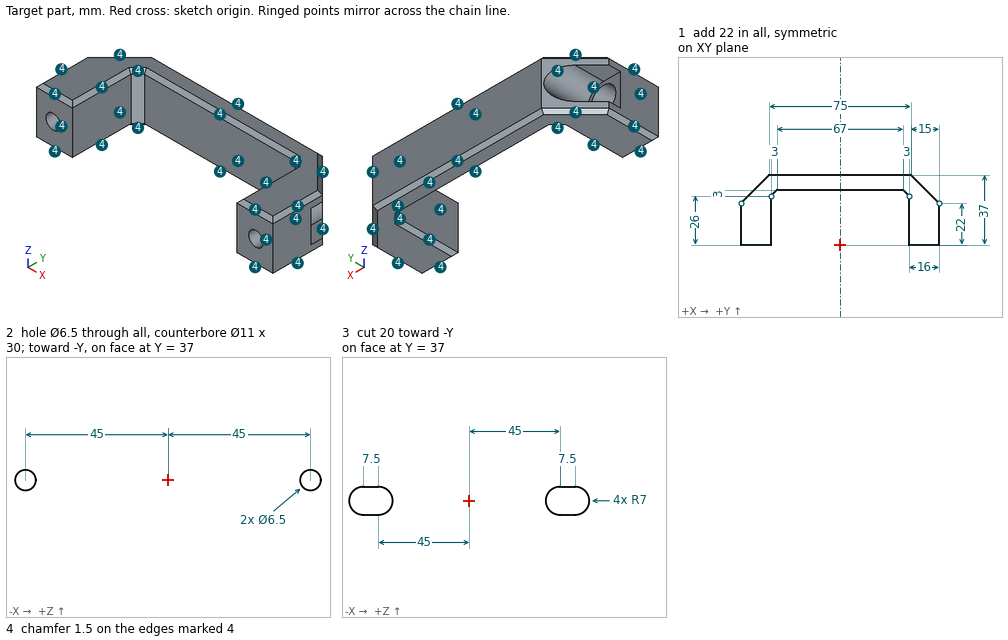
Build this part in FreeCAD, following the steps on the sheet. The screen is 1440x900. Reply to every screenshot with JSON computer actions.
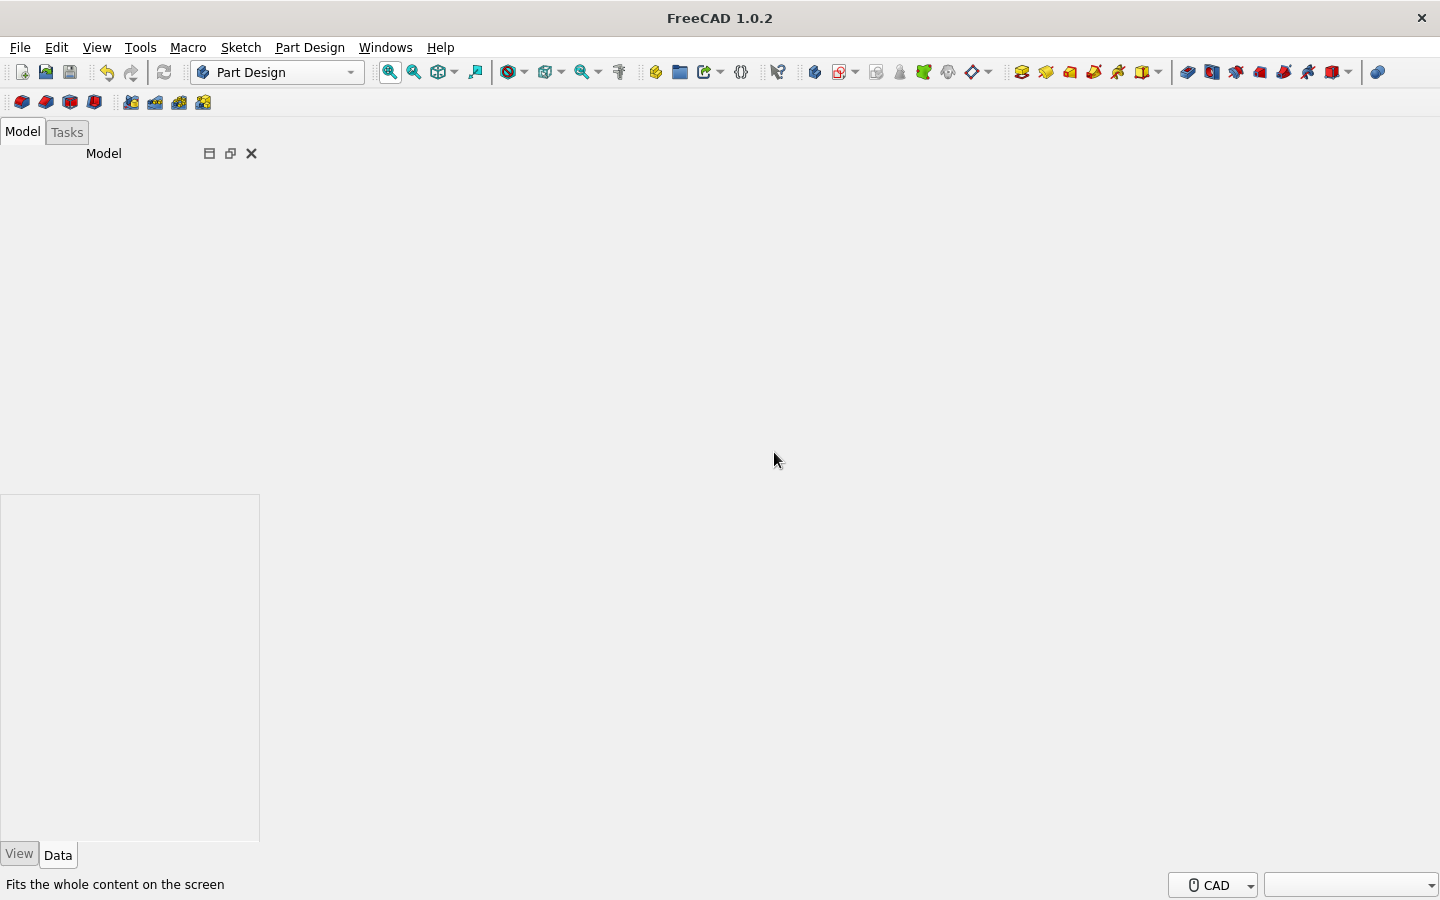
{"action": "left_click", "coordinate": [22, 72]}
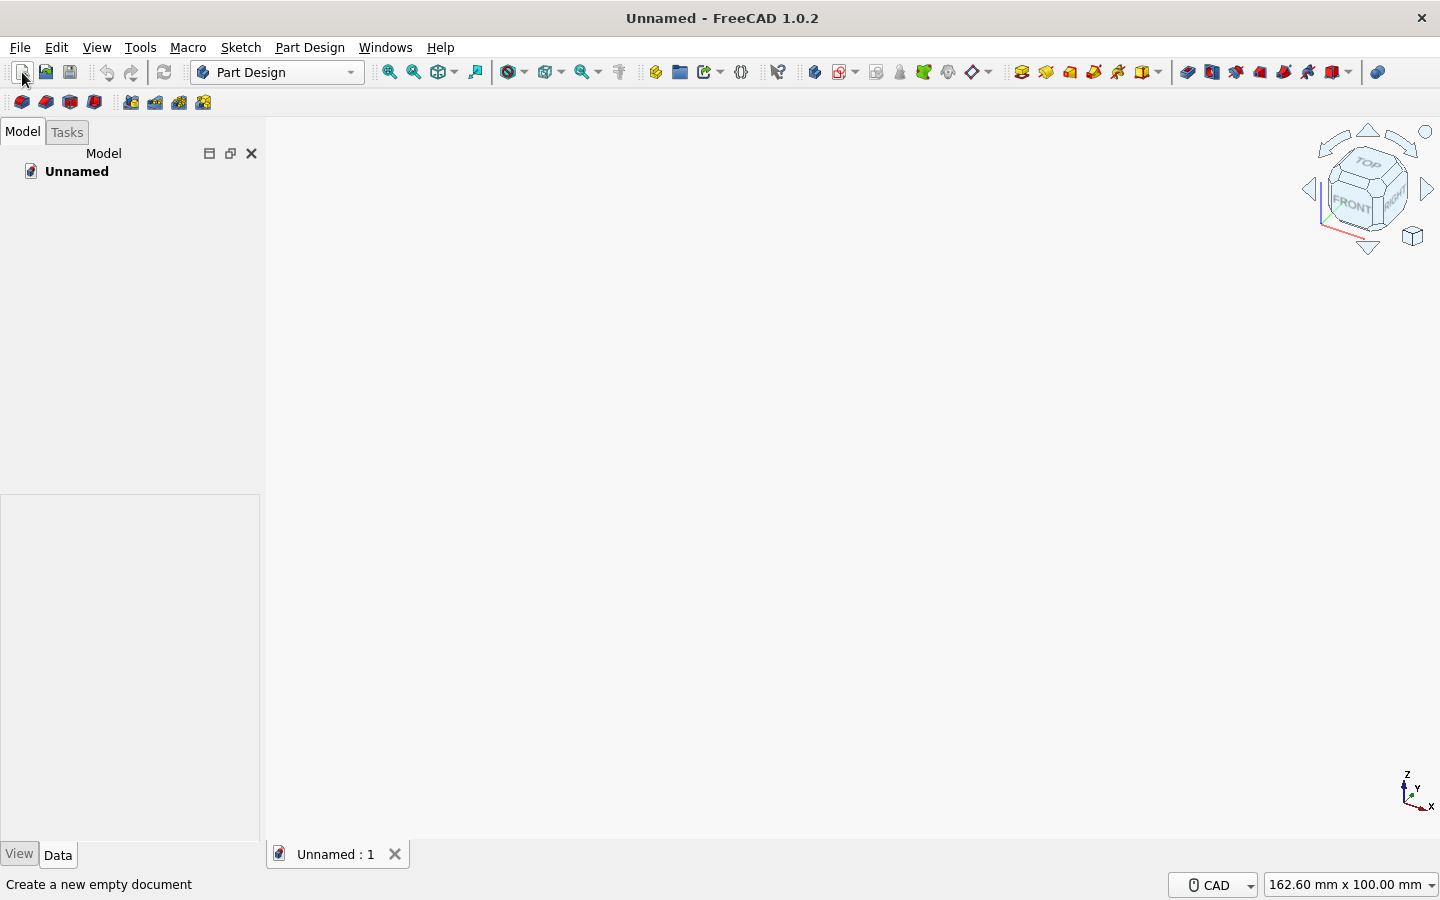
{"action": "left_click", "coordinate": [840, 72]}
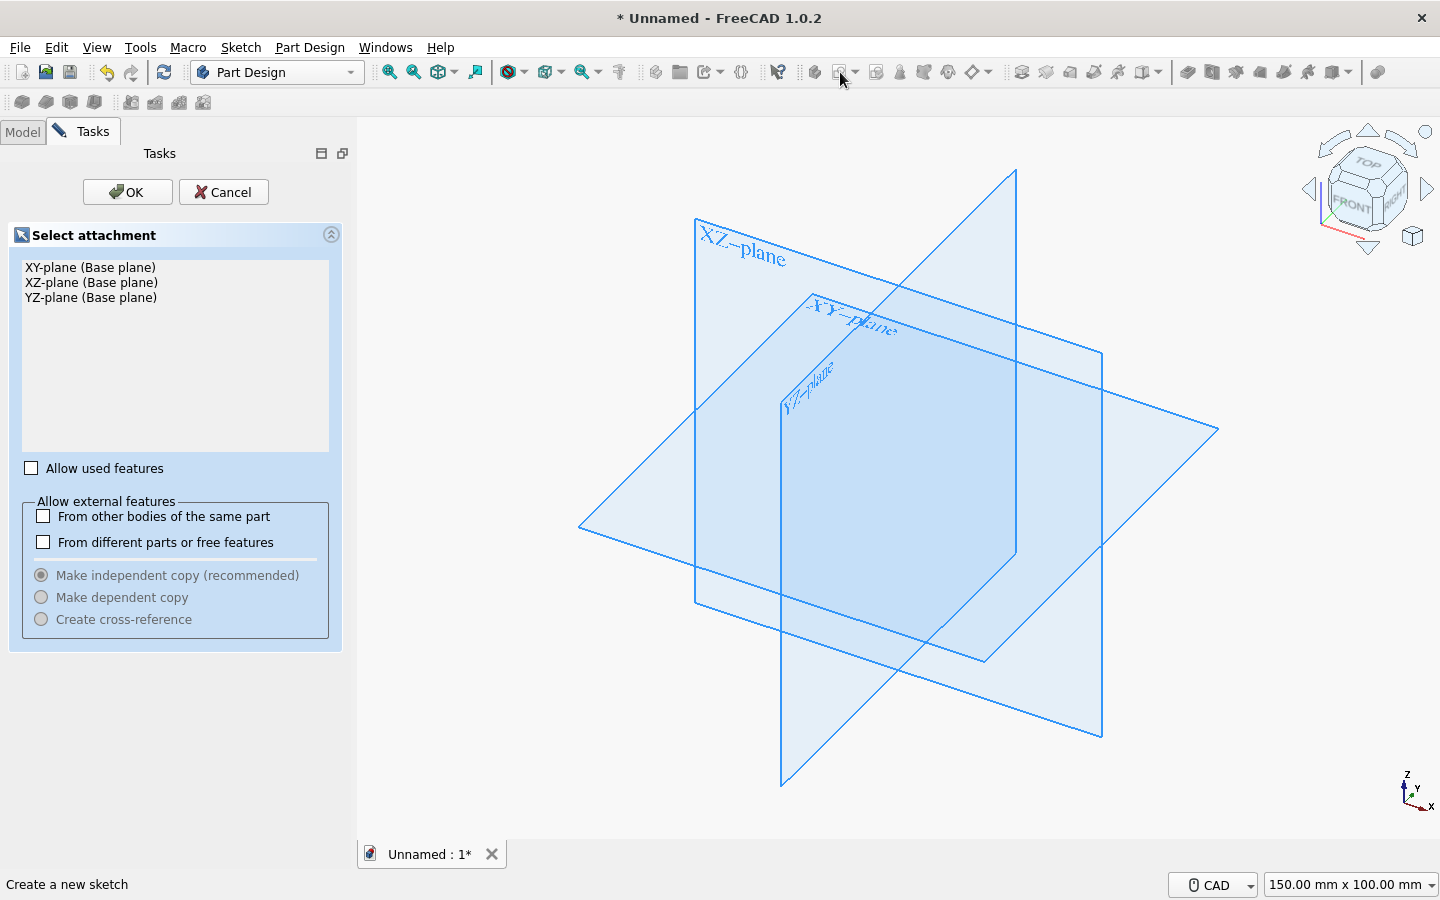
{"action": "left_click", "coordinate": [82, 268]}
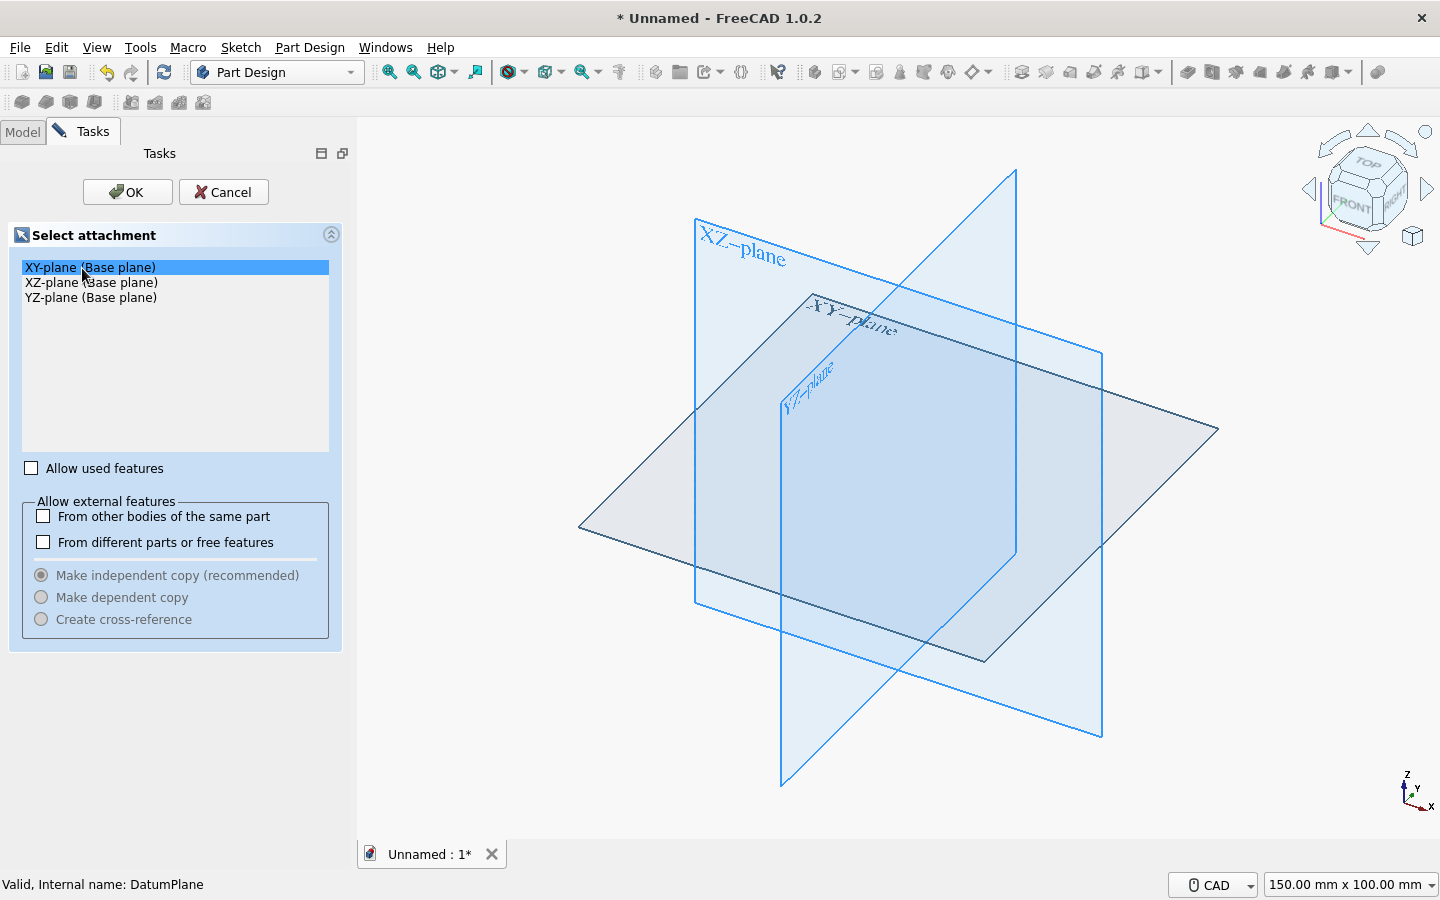
{"action": "left_click", "coordinate": [128, 192]}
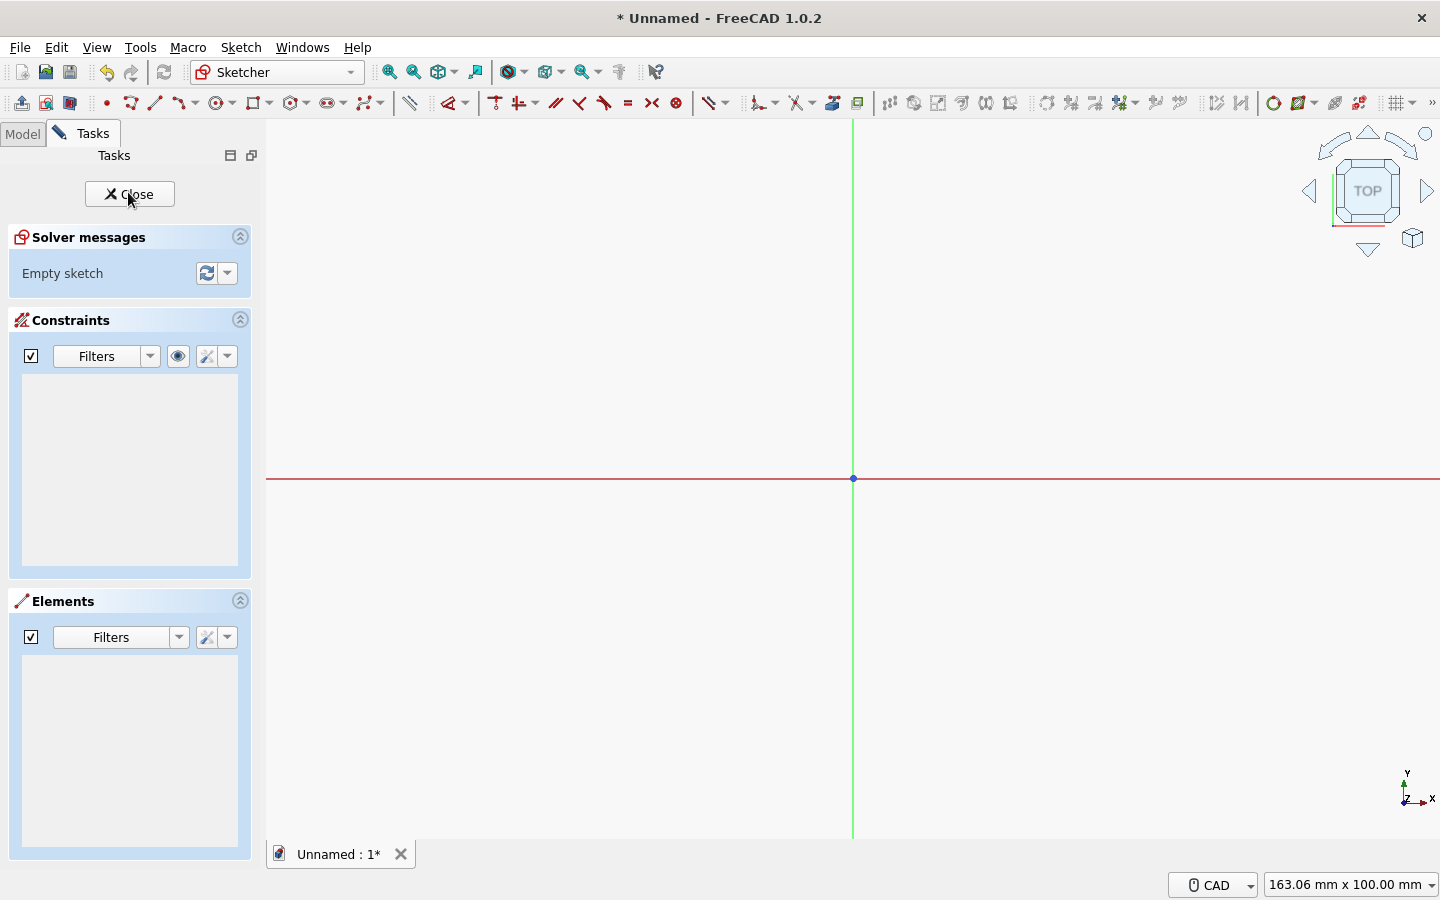
{"action": "left_click", "coordinate": [132, 104]}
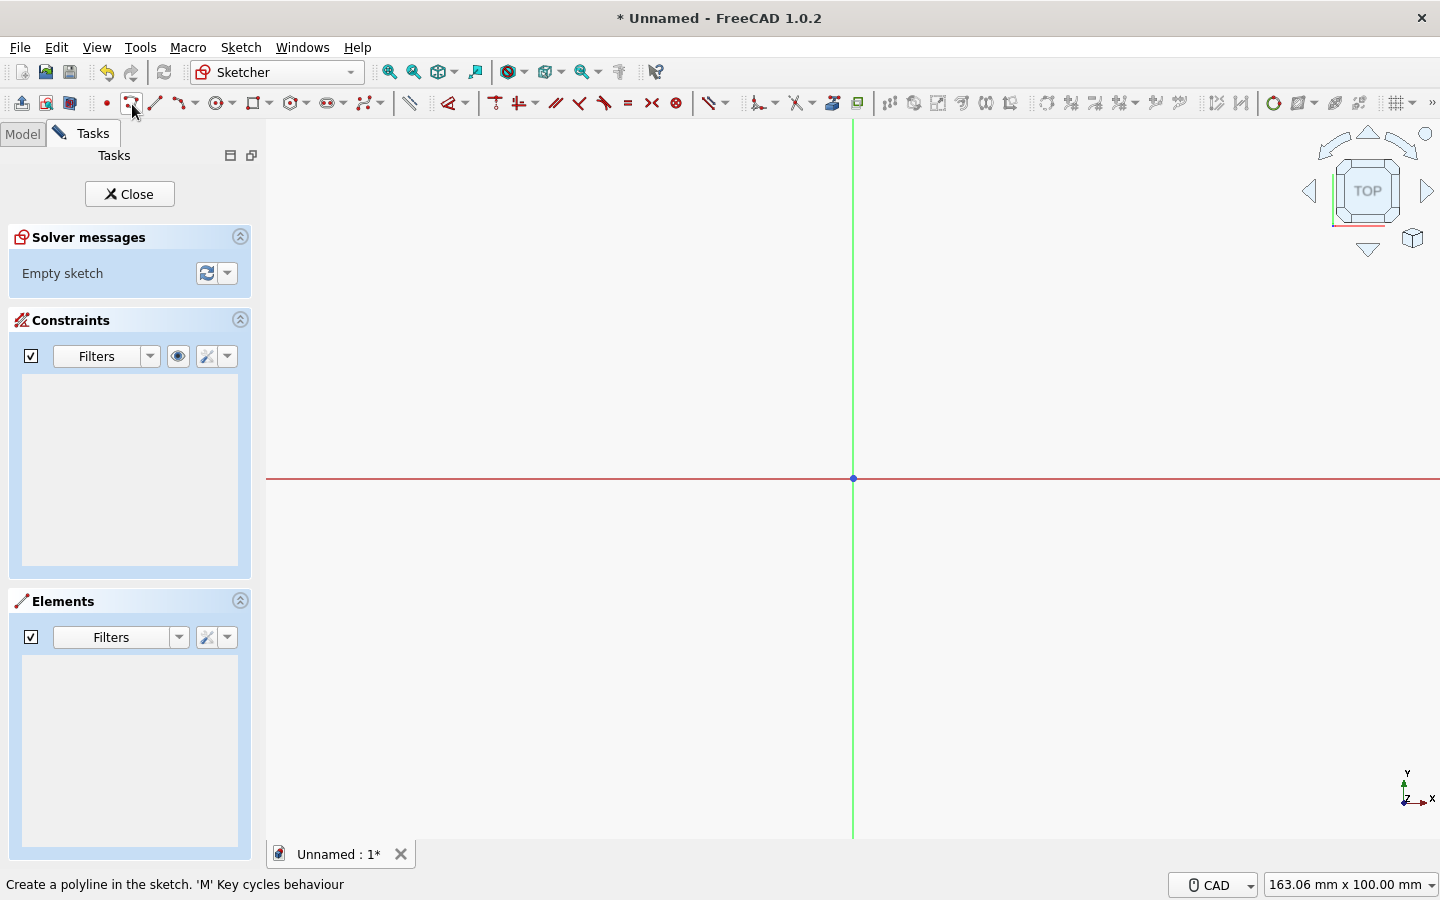
{"action": "left_click", "coordinate": [590, 479]}
{"action": "left_click", "coordinate": [590, 292]}
{"action": "left_click", "coordinate": [612, 270]}
{"action": "left_click", "coordinate": [1094, 270]}
{"action": "left_click", "coordinate": [1116, 292]}
{"action": "left_click", "coordinate": [1116, 479]}
{"action": "left_click", "coordinate": [1231, 470]}
{"action": "left_click", "coordinate": [1231, 321]}
{"action": "left_click", "coordinate": [1123, 213]}
{"action": "left_click", "coordinate": [583, 213]}
{"action": "left_click", "coordinate": [475, 321]}
{"action": "left_click", "coordinate": [475, 470]}
{"action": "left_click", "coordinate": [590, 479]}
{"action": "key", "text": "Escape"}
{"action": "key", "text": "Escape"}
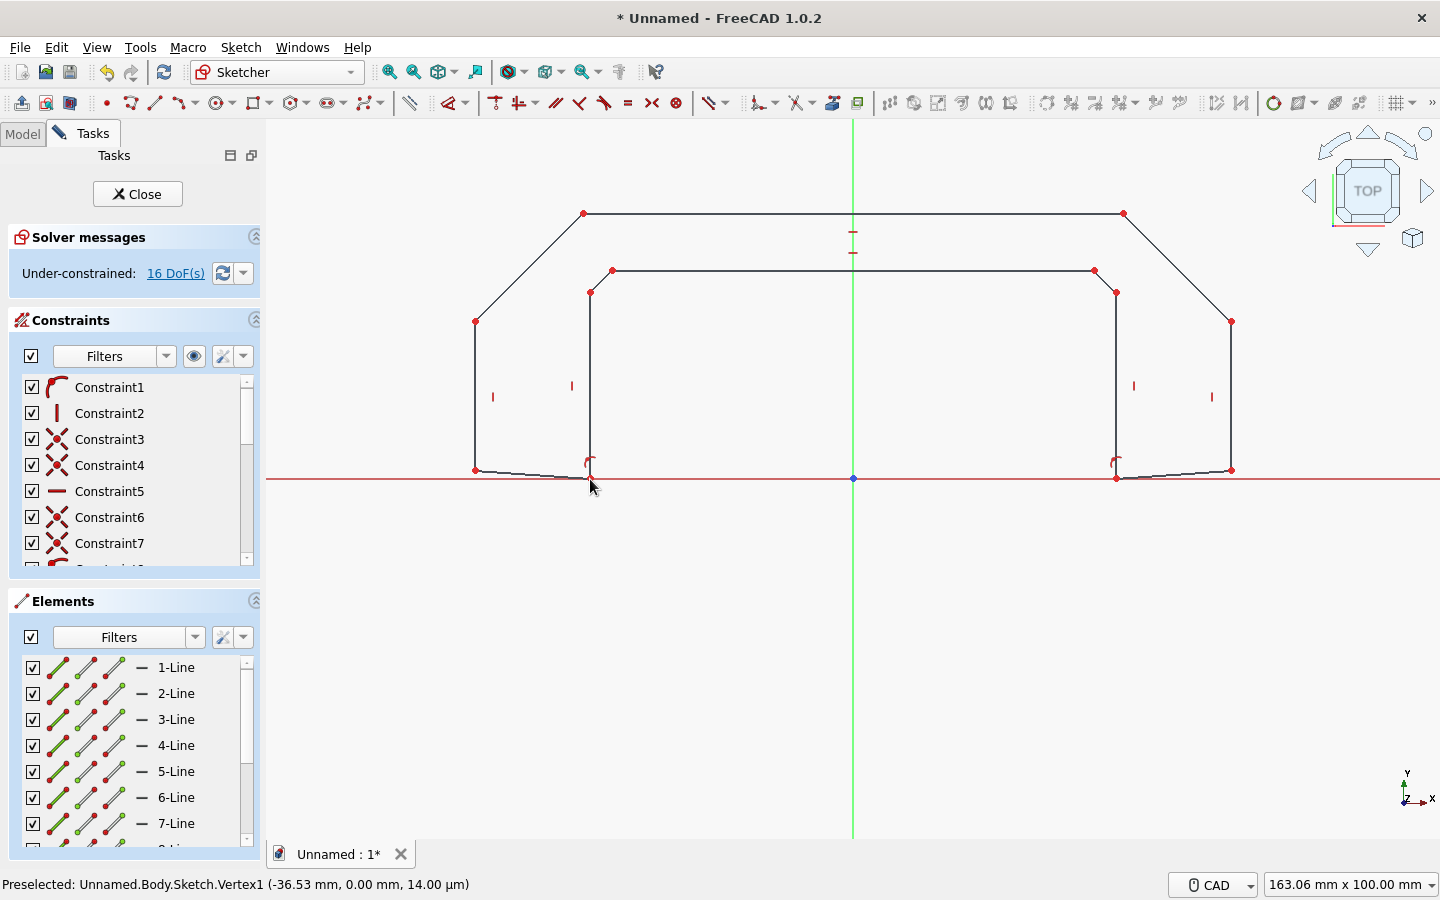
{"action": "left_click", "coordinate": [1150, 477]}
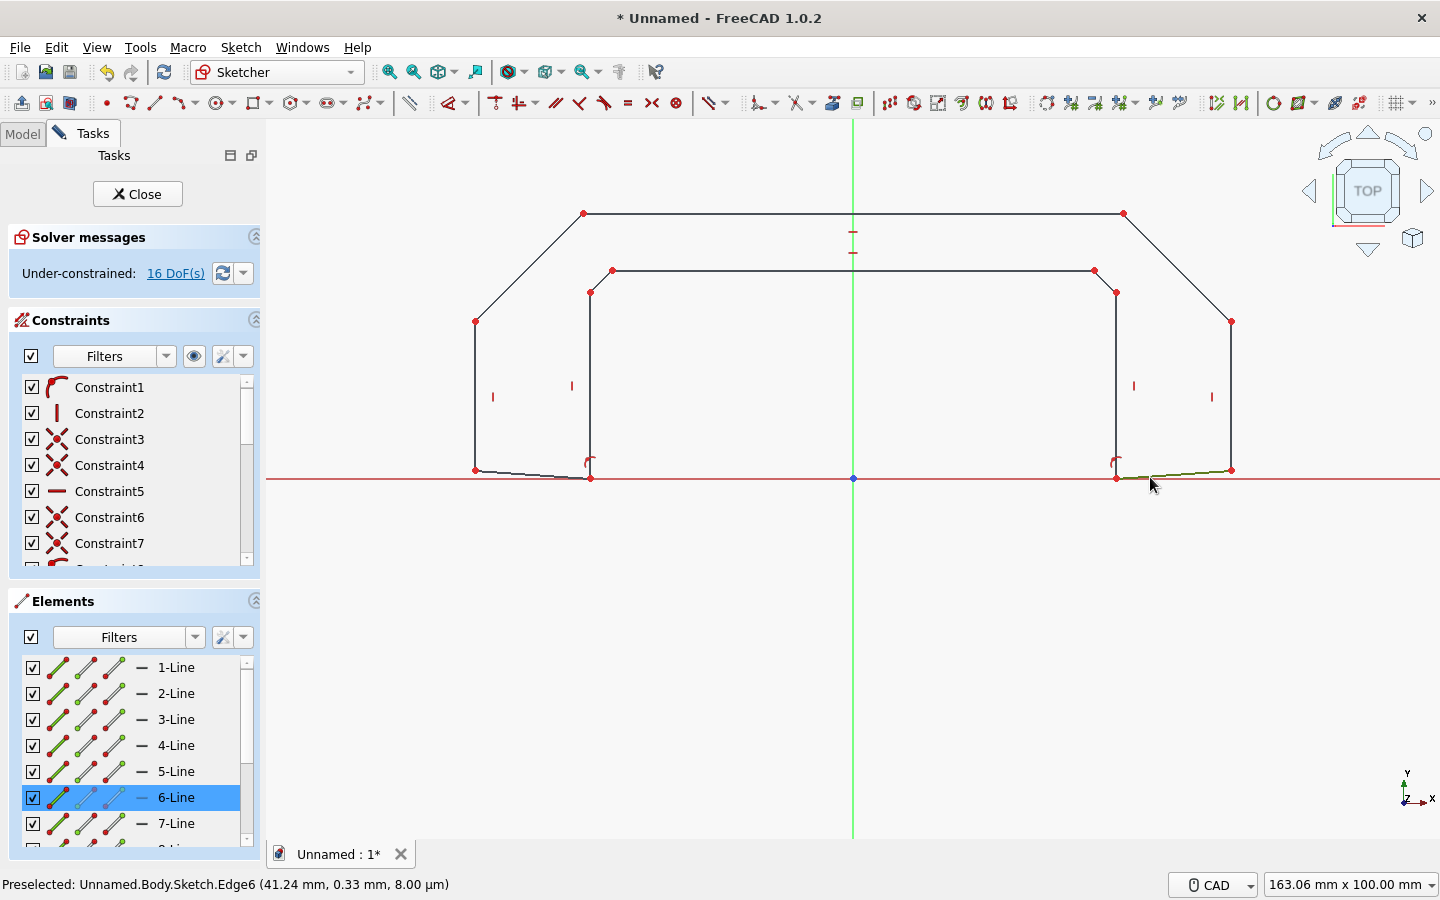
{"action": "left_click", "coordinate": [538, 104]}